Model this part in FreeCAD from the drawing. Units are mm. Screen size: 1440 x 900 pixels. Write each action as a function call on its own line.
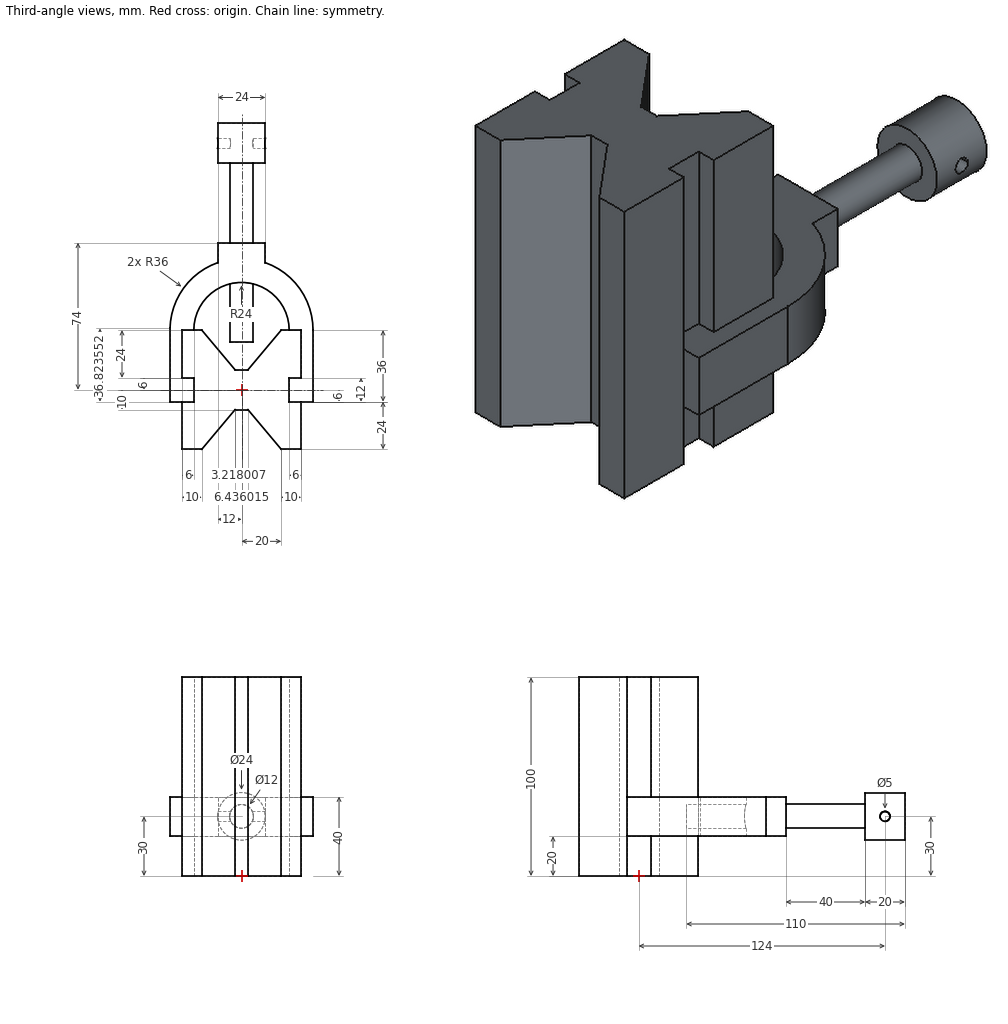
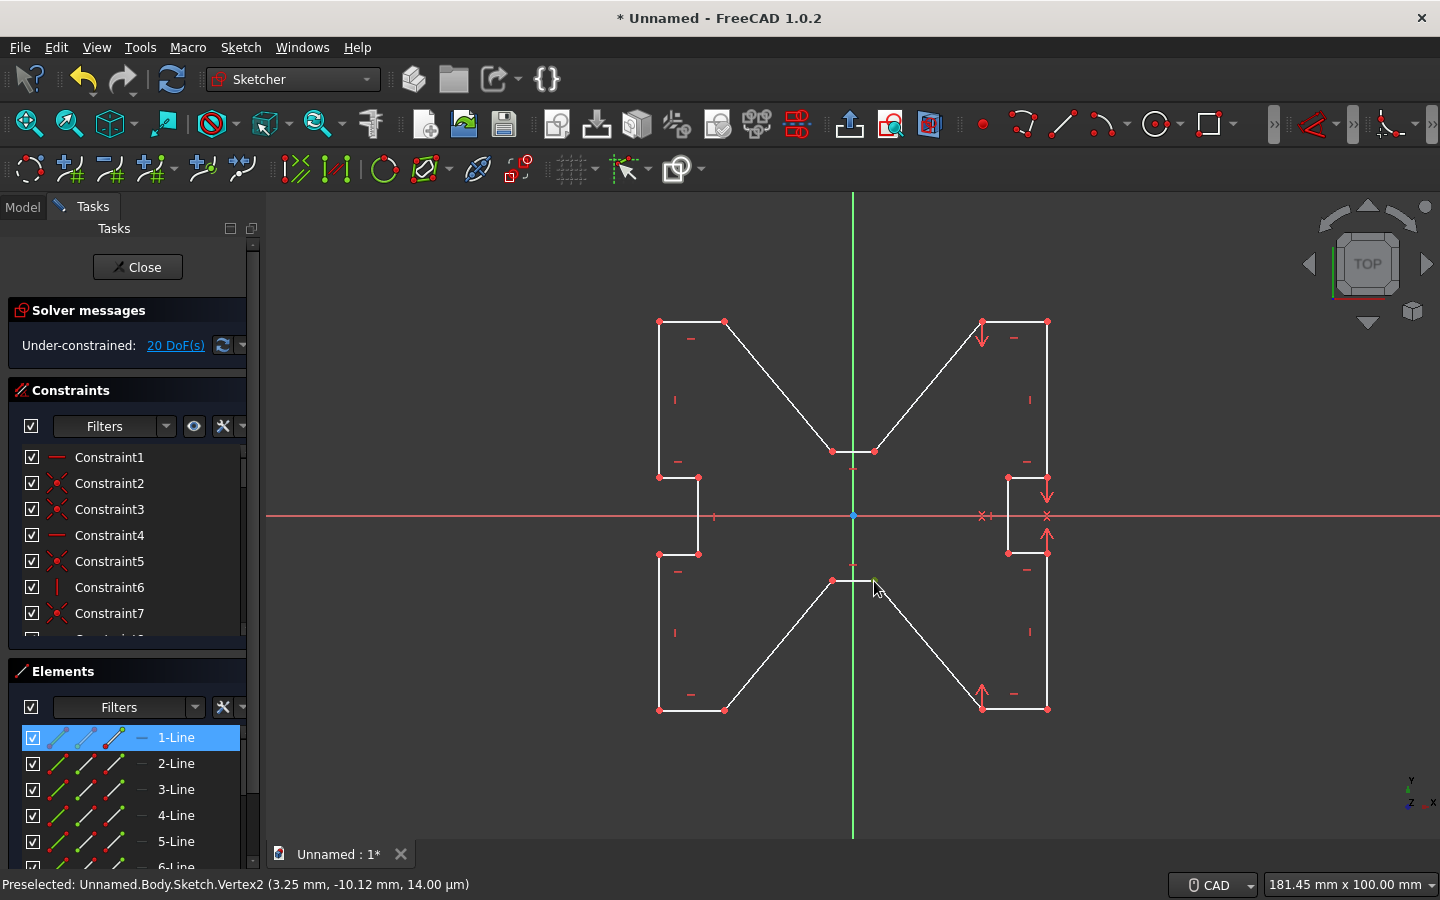
click(874, 452)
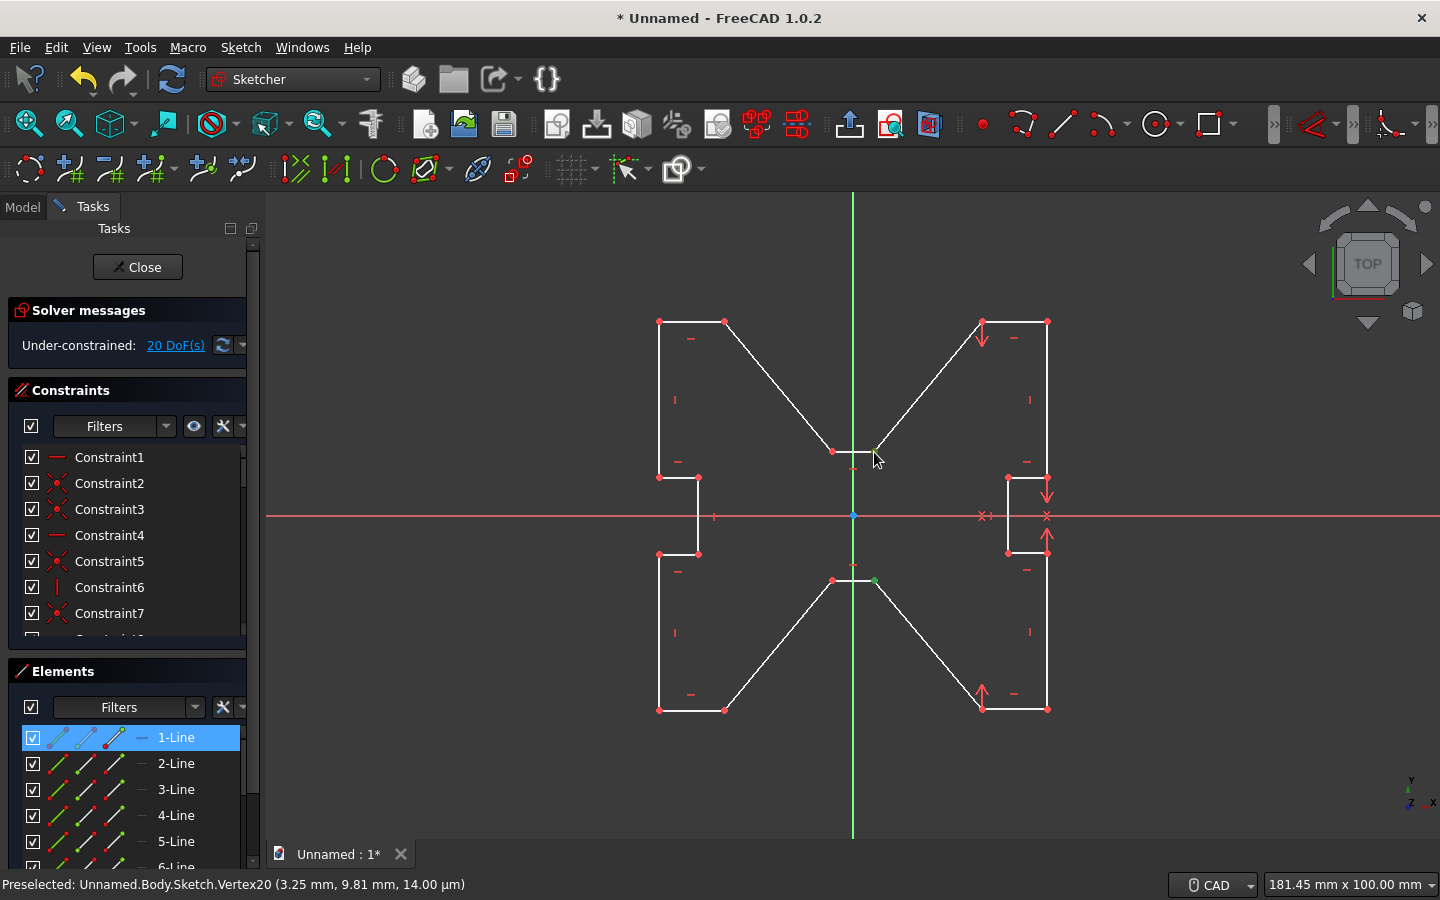
click(364, 516)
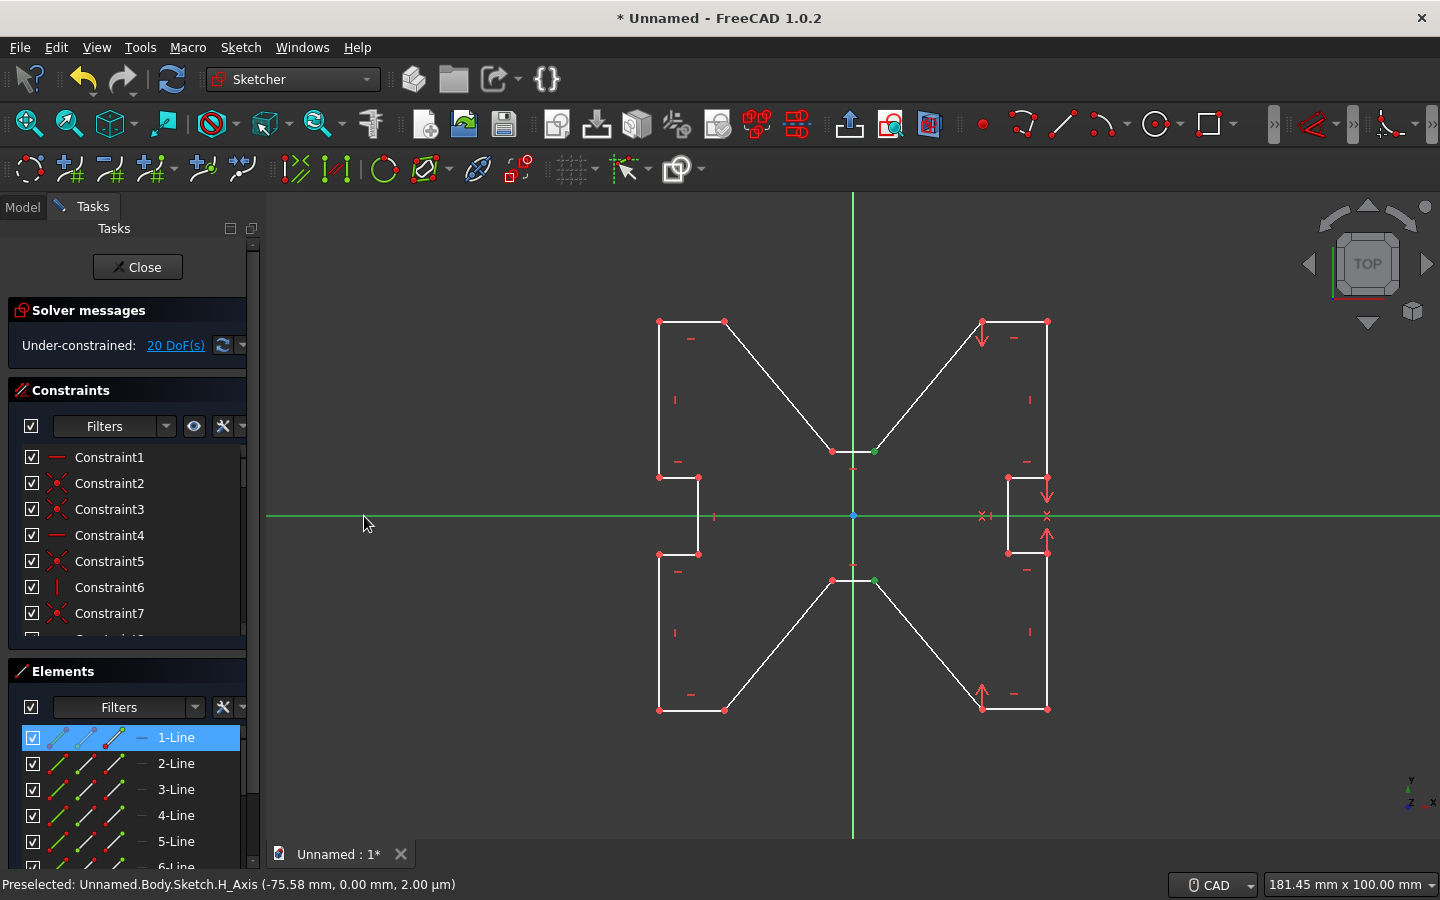
key(s)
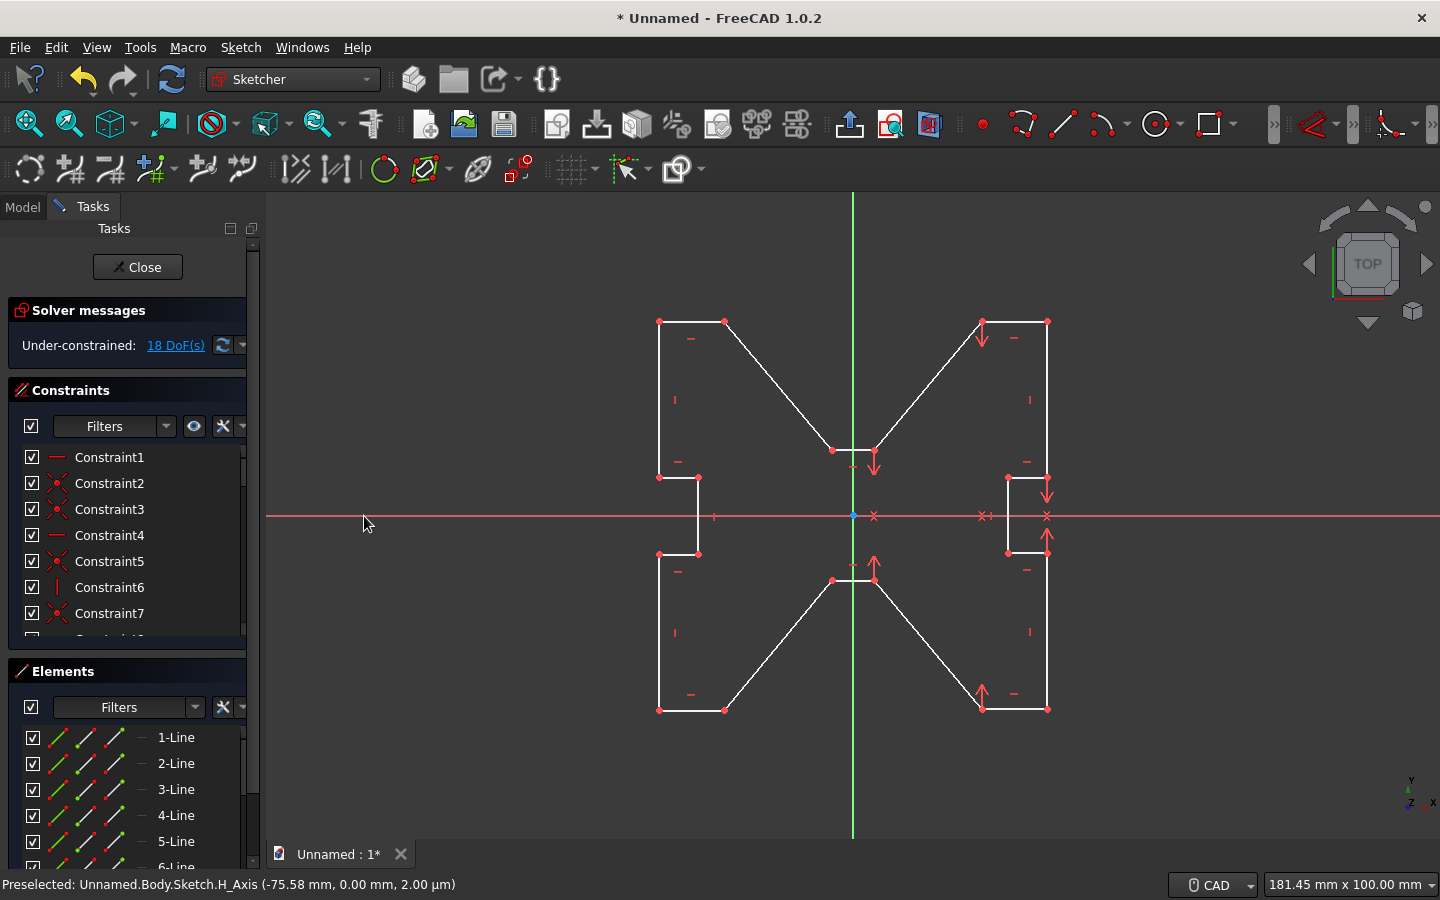
click(982, 322)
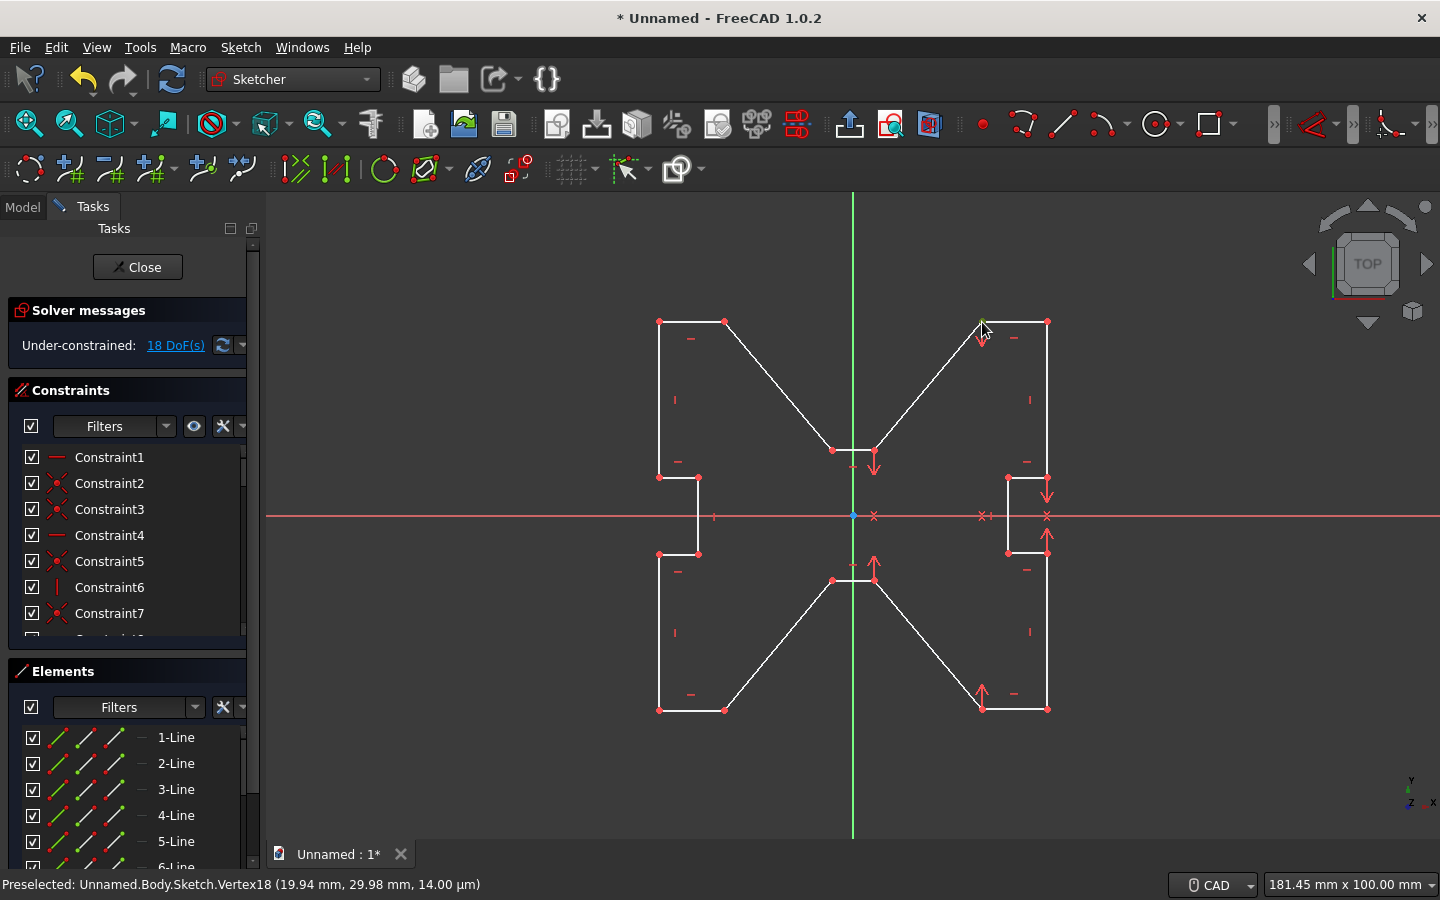
click(724, 322)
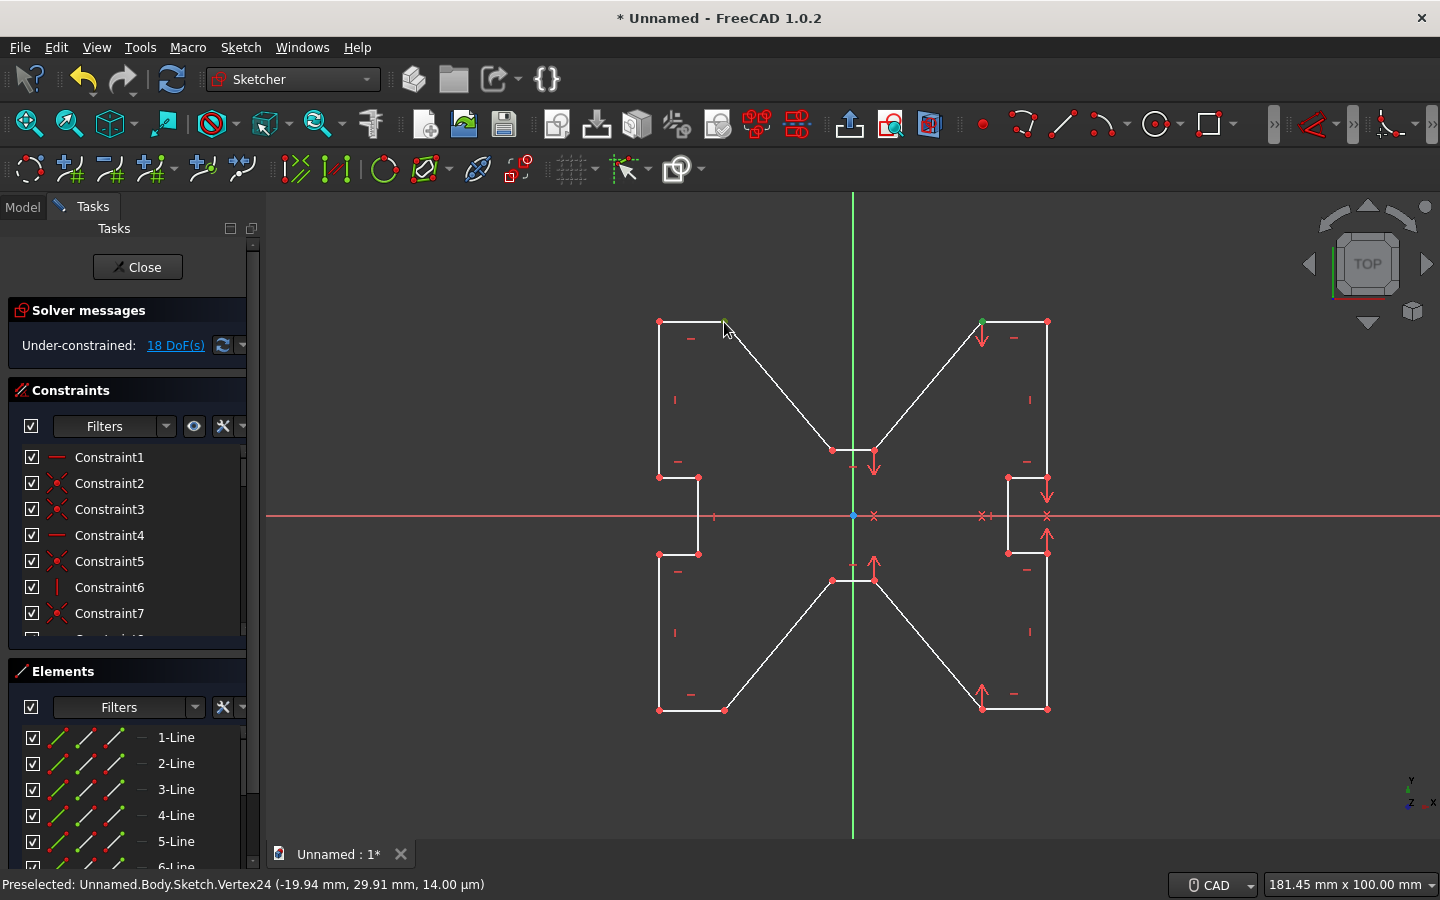
click(853, 769)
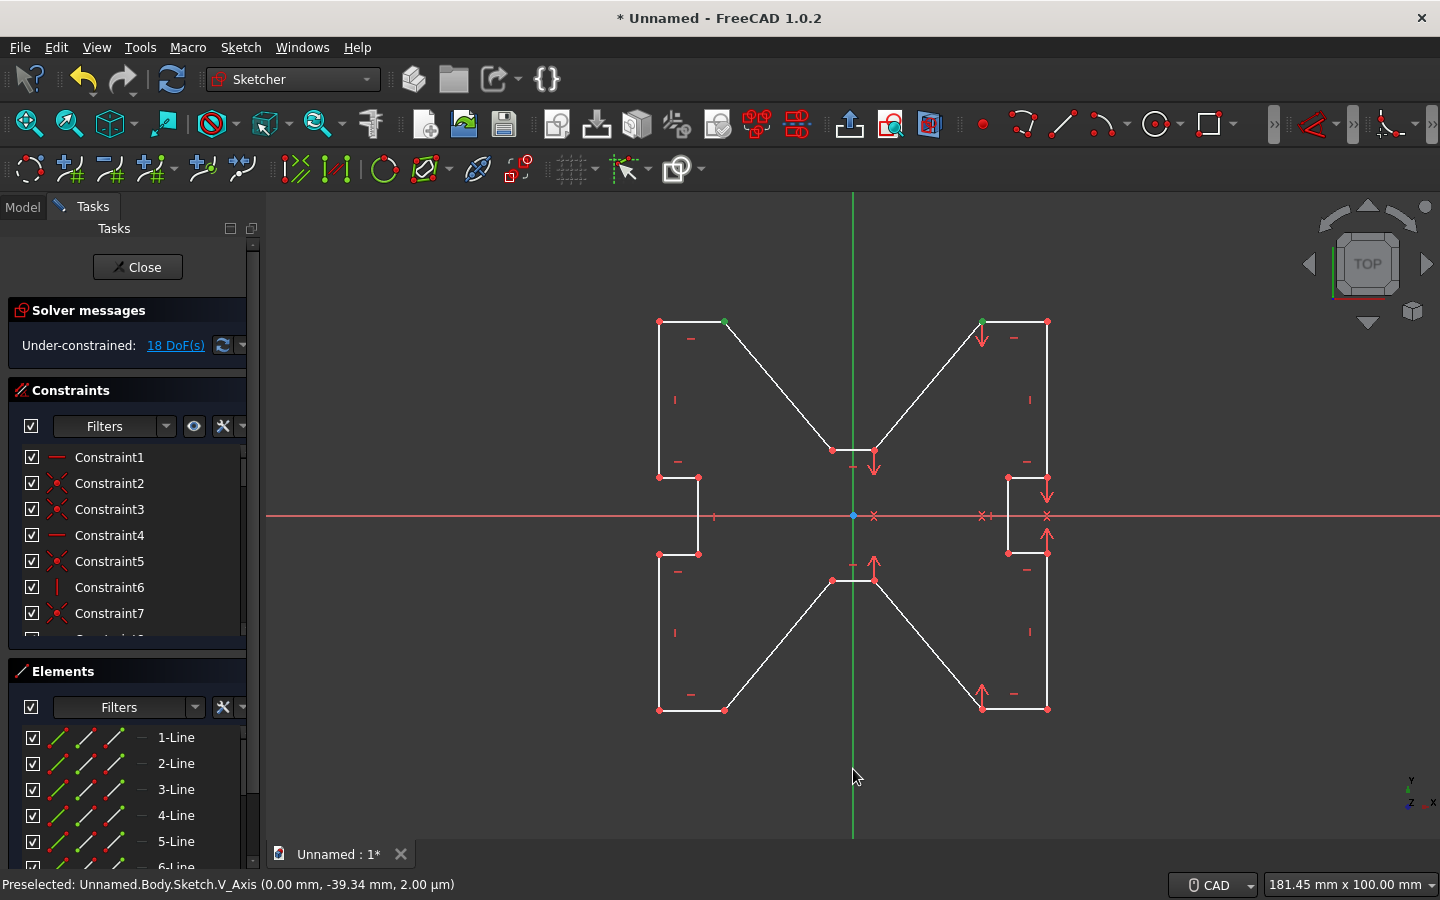
key(s)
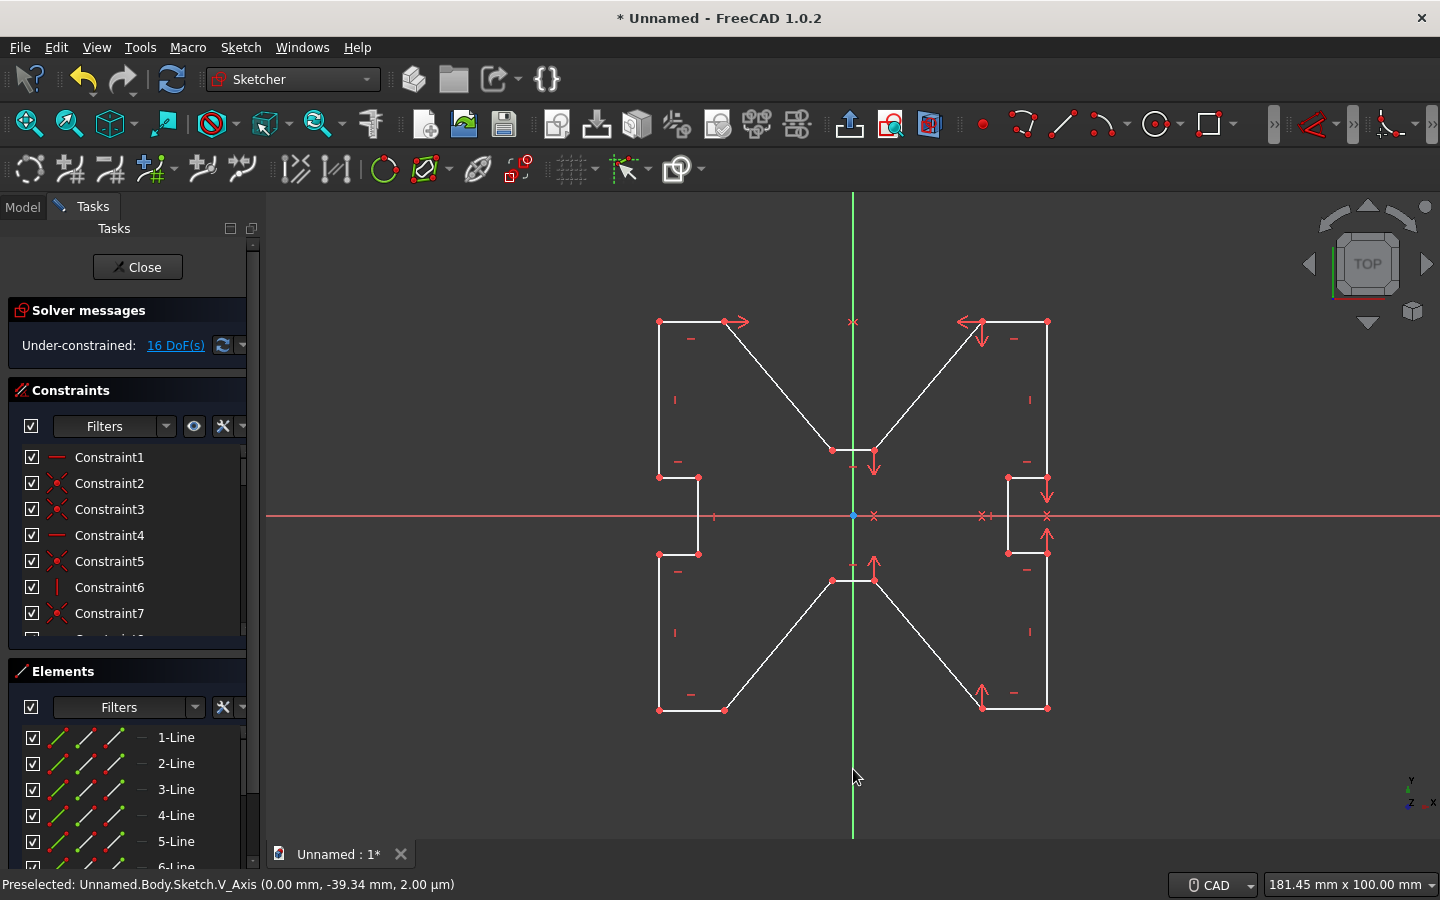
click(1047, 478)